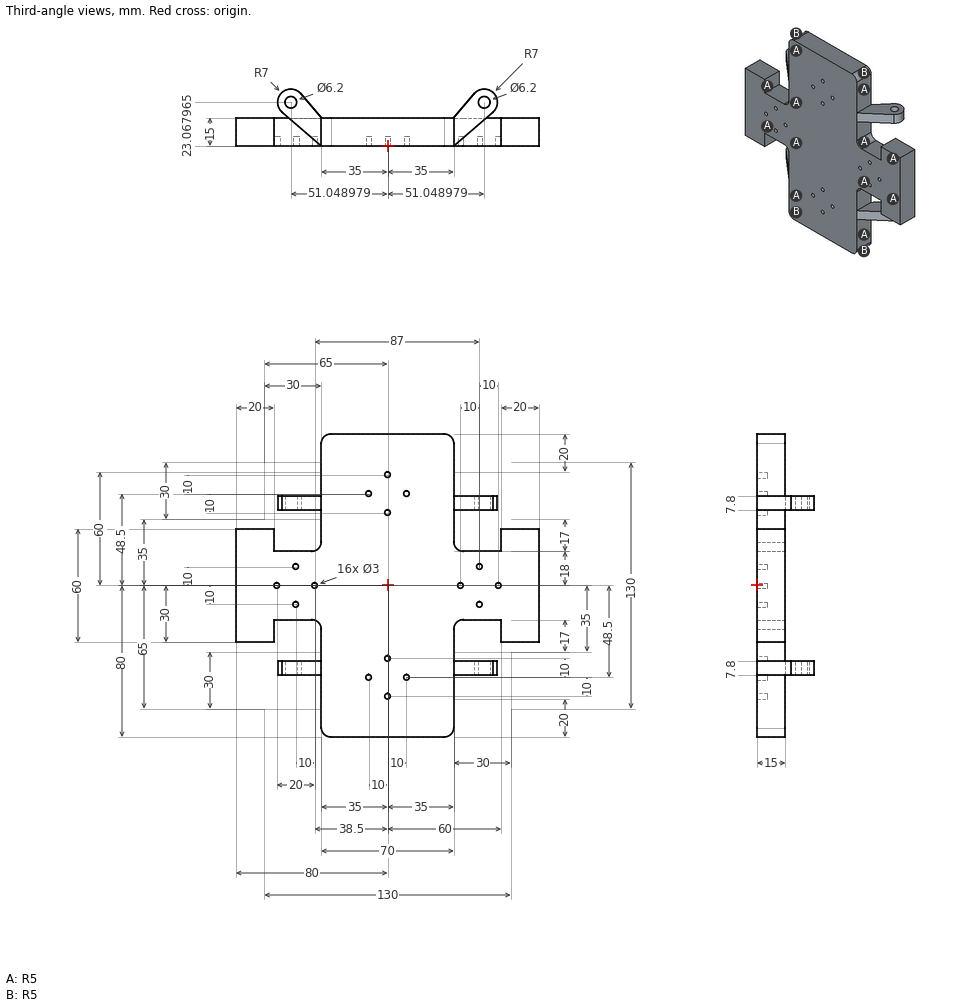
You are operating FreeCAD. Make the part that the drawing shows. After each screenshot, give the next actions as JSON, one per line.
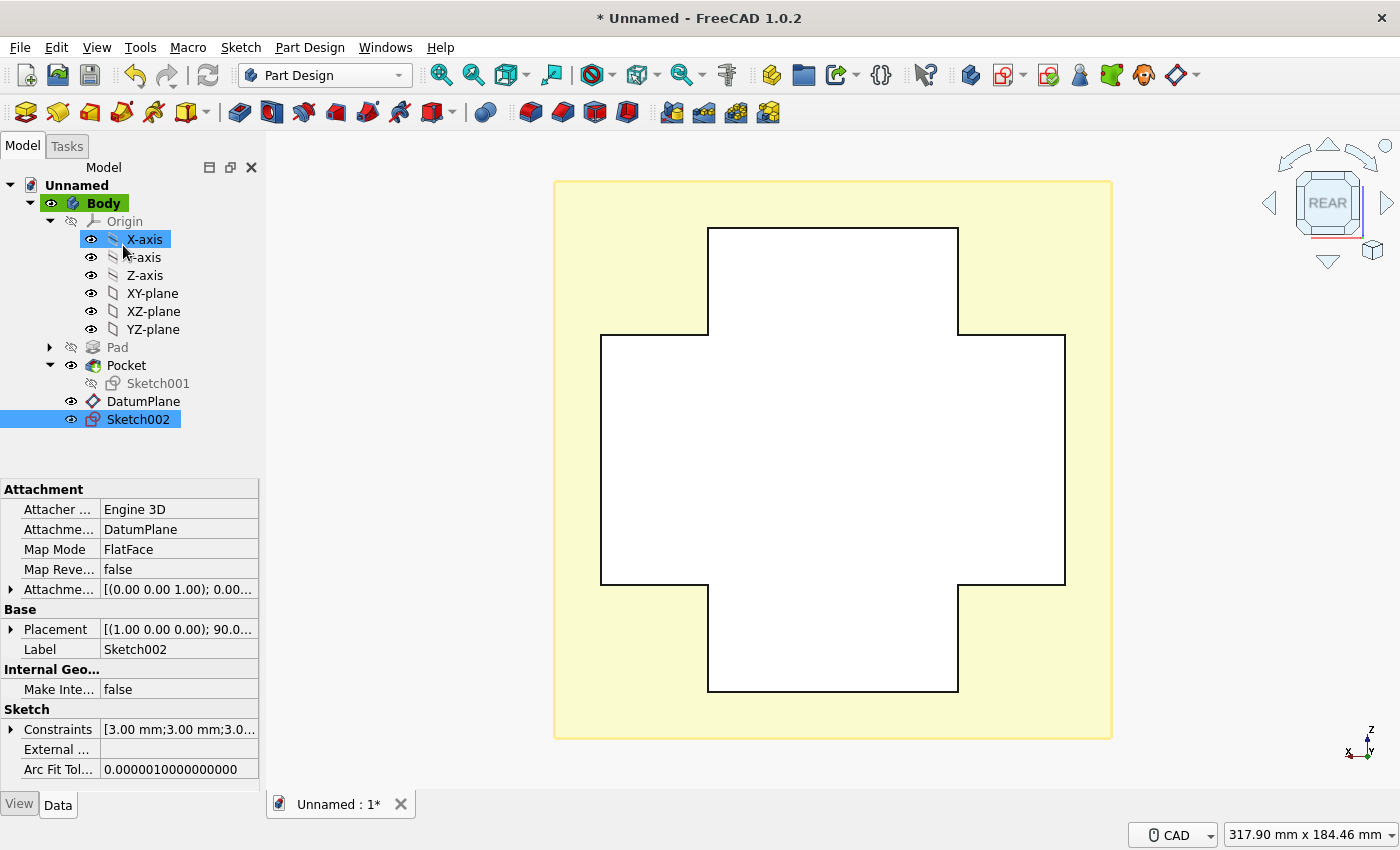
{"action": "left_click", "coordinate": [240, 112]}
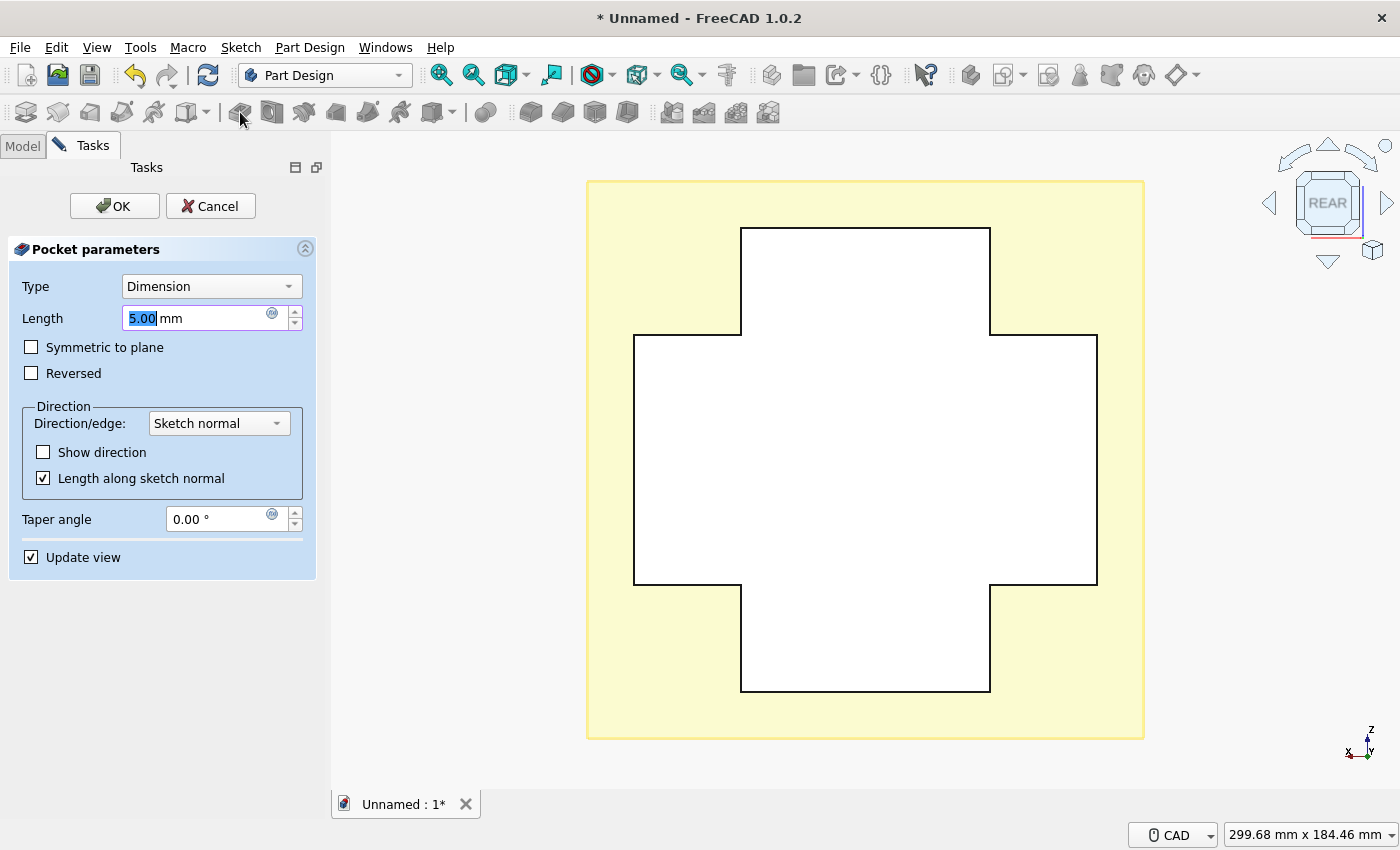
{"action": "left_click", "coordinate": [212, 286]}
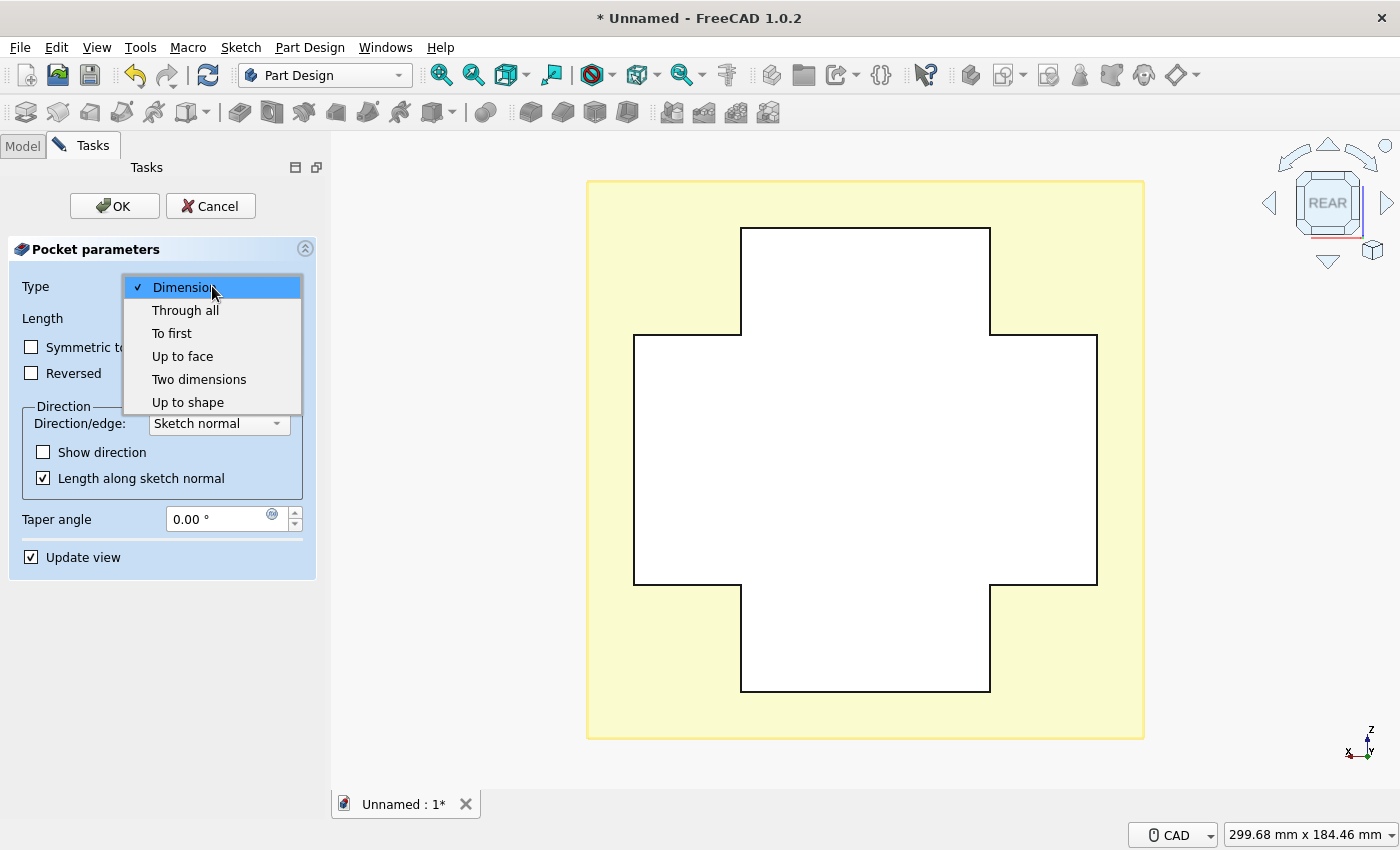
{"action": "left_click", "coordinate": [212, 310]}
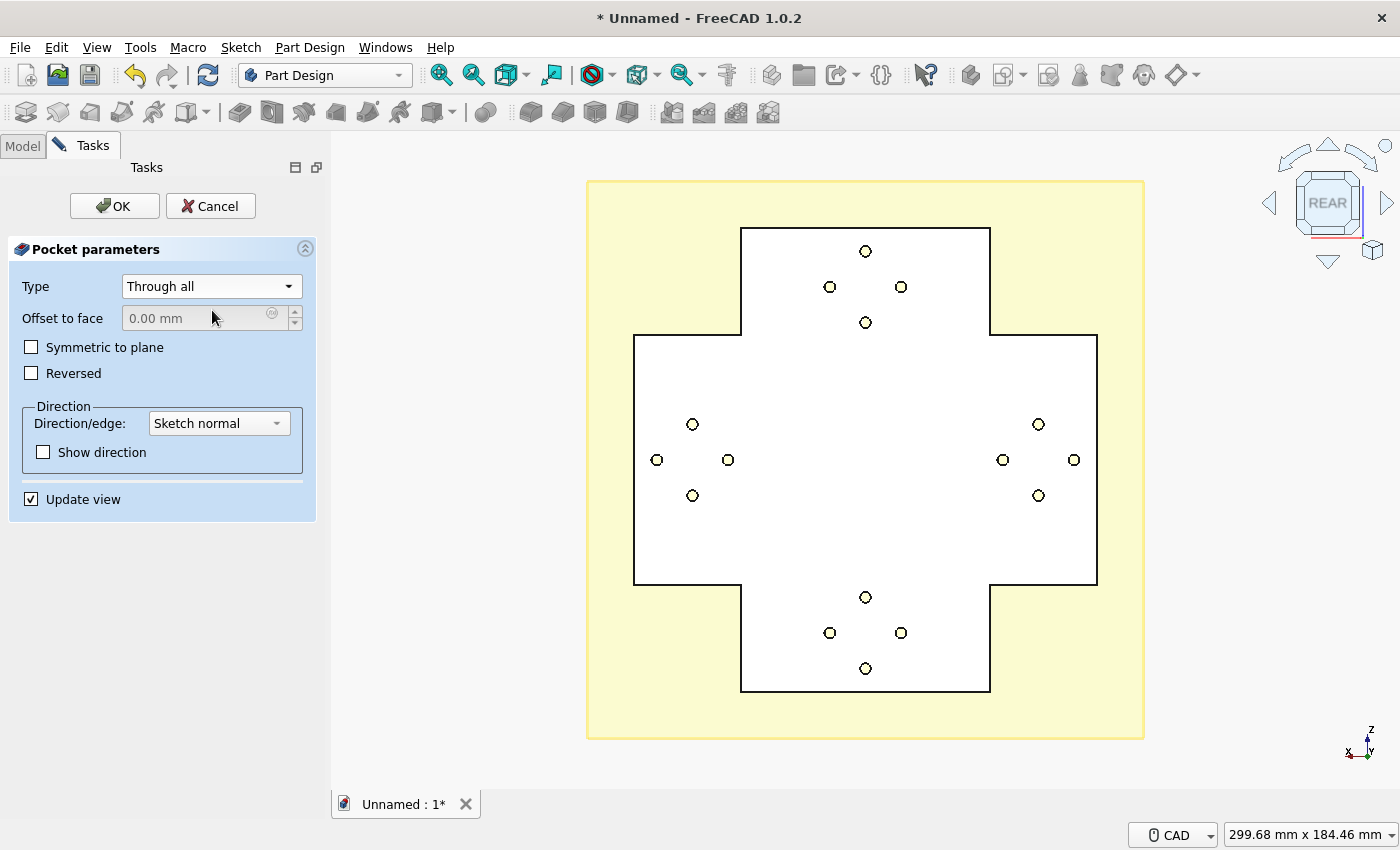
{"action": "left_click", "coordinate": [30, 373]}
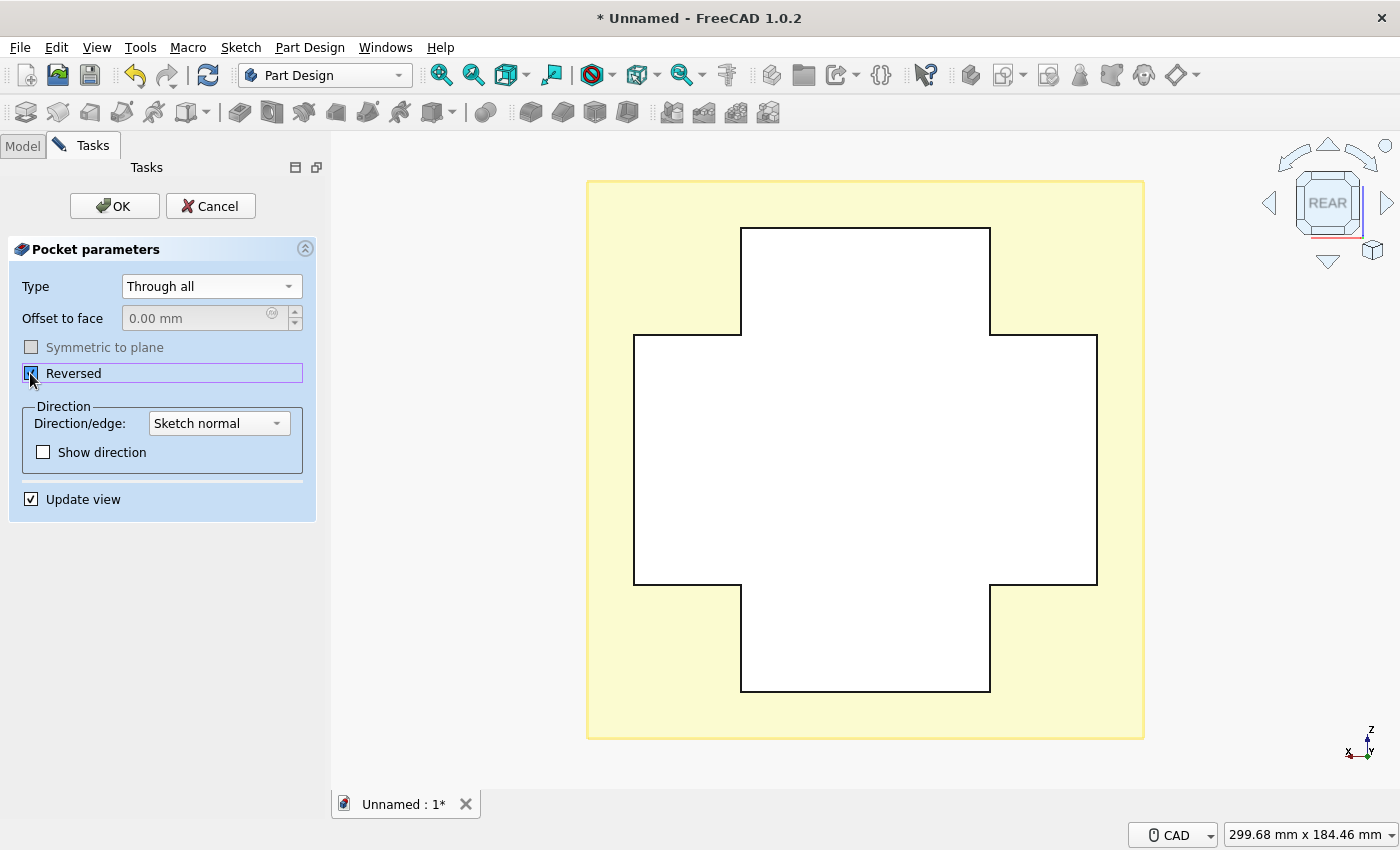
{"action": "left_click", "coordinate": [115, 206]}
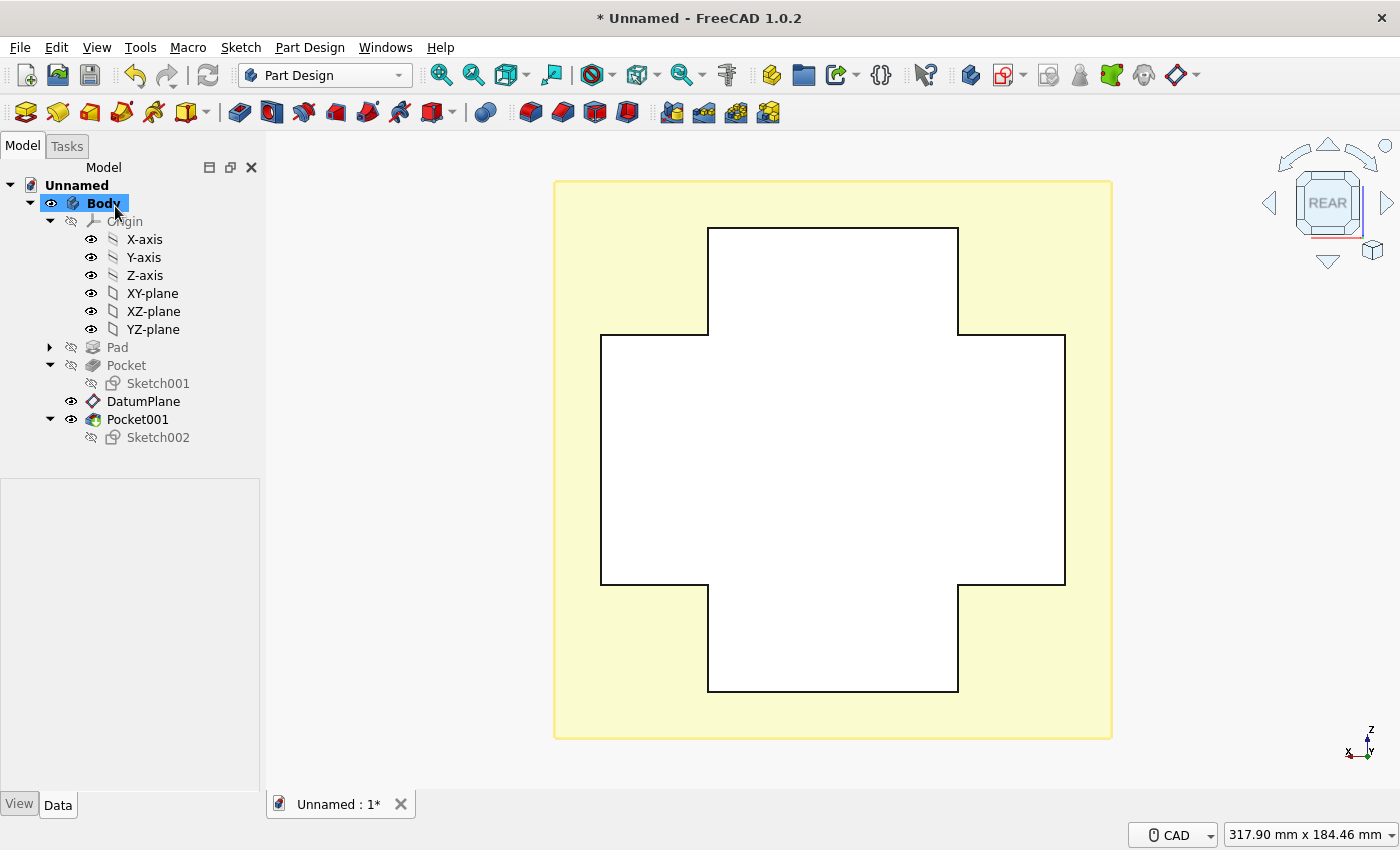
{"action": "left_click", "coordinate": [116, 401]}
{"action": "key", "text": "space"}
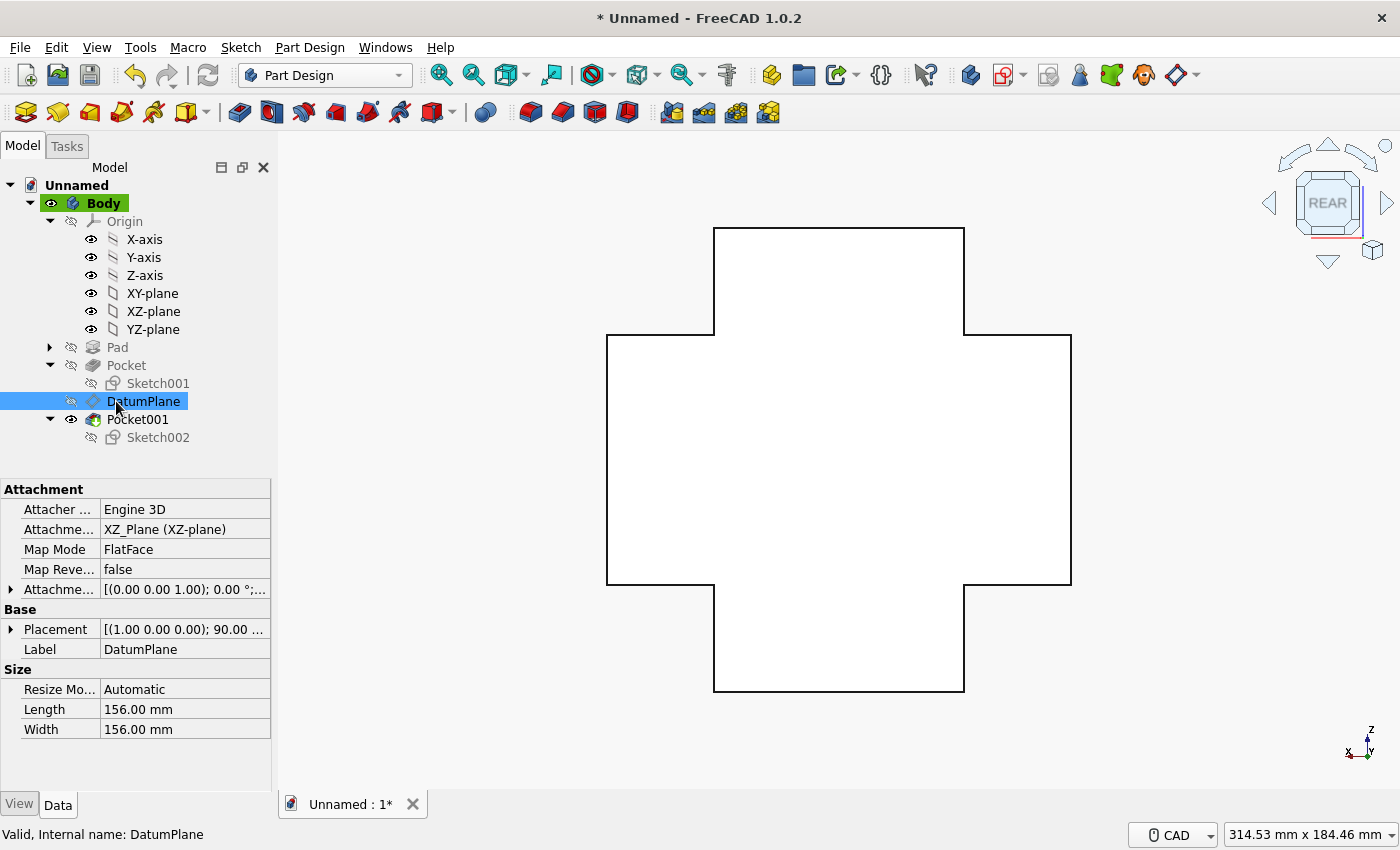
{"action": "left_click", "coordinate": [839, 459]}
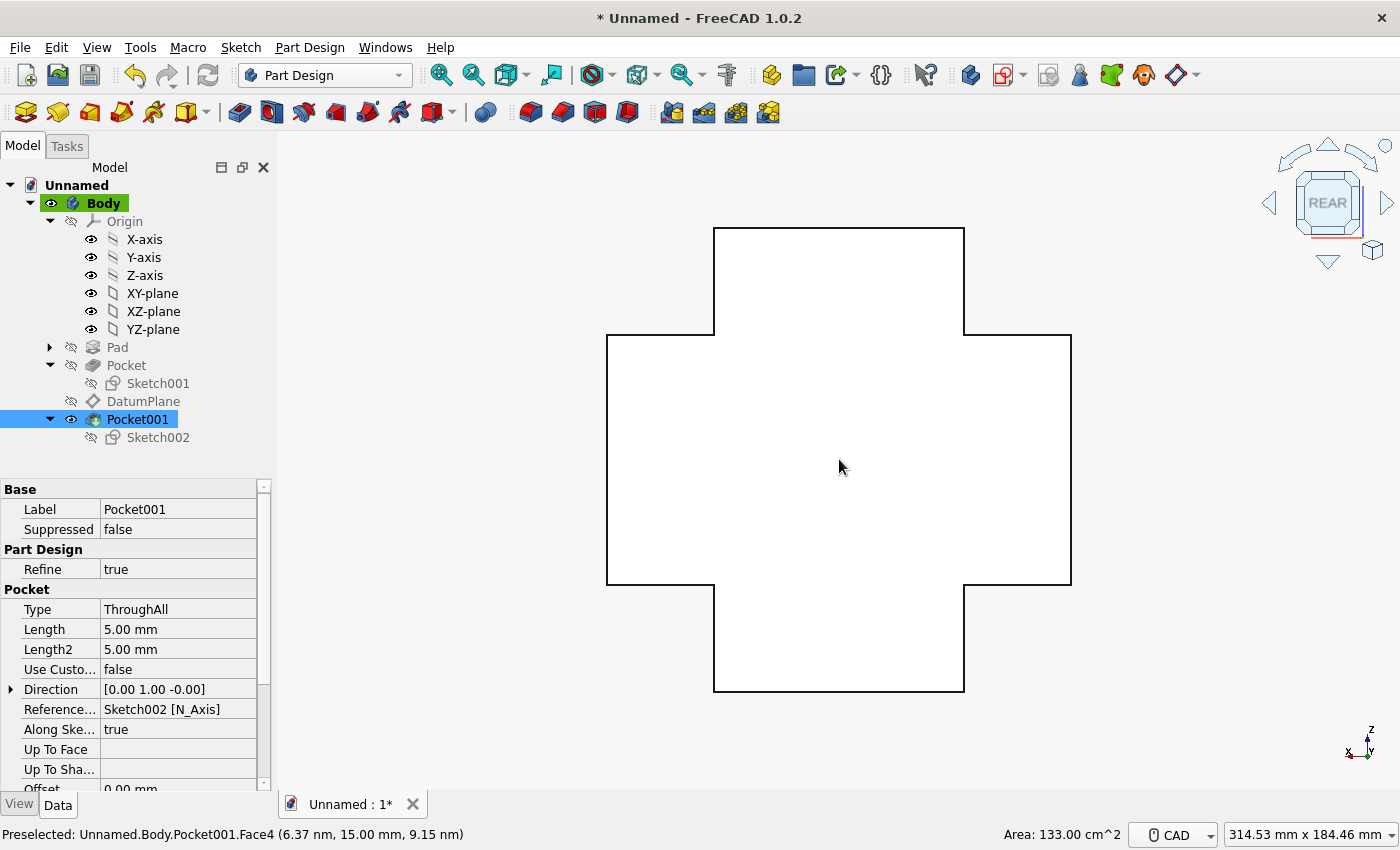
{"action": "left_click", "coordinate": [1004, 76]}